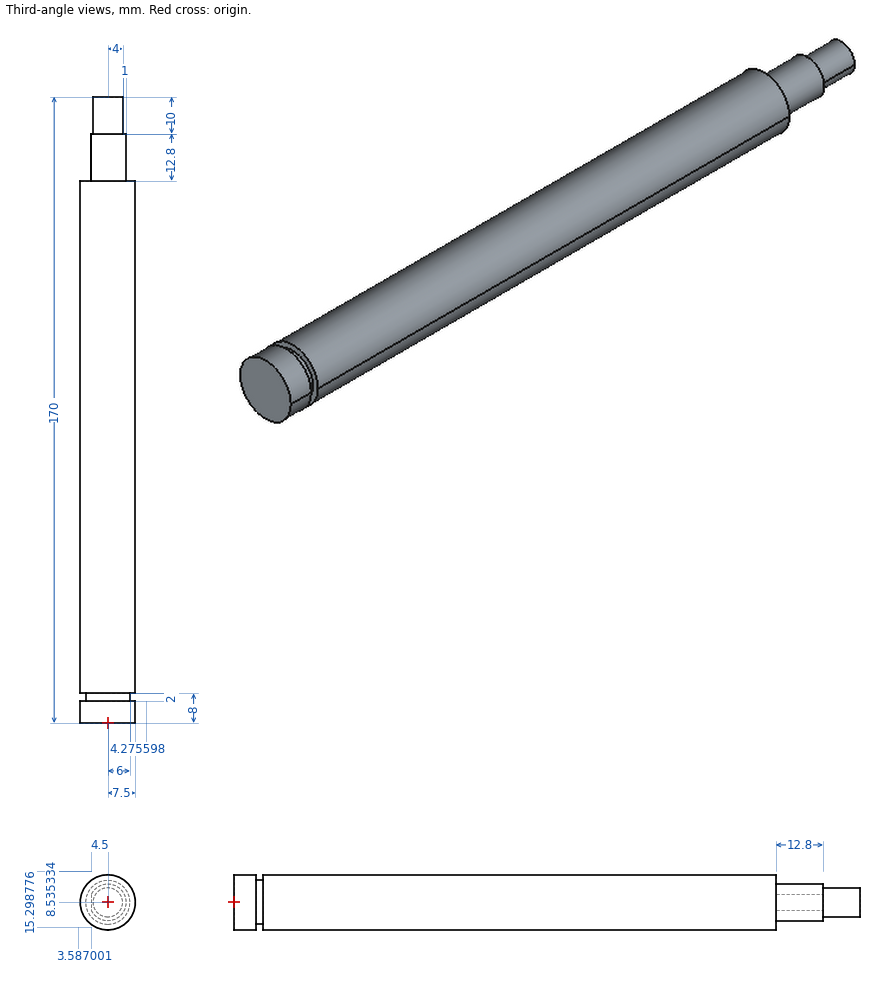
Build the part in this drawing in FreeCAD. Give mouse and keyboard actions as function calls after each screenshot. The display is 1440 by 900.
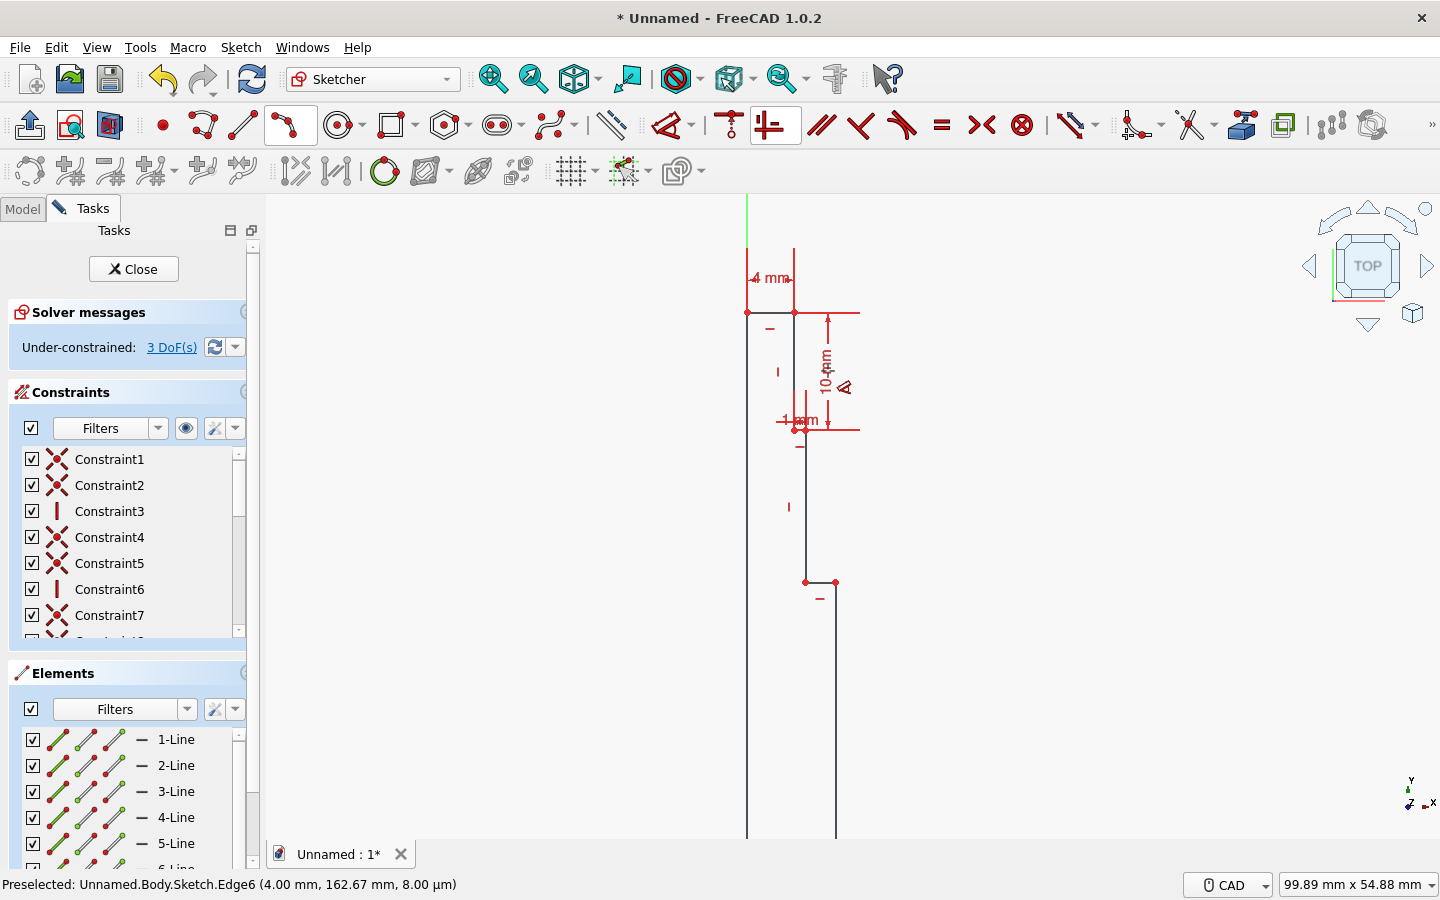
scroll(783, 316, down, 8)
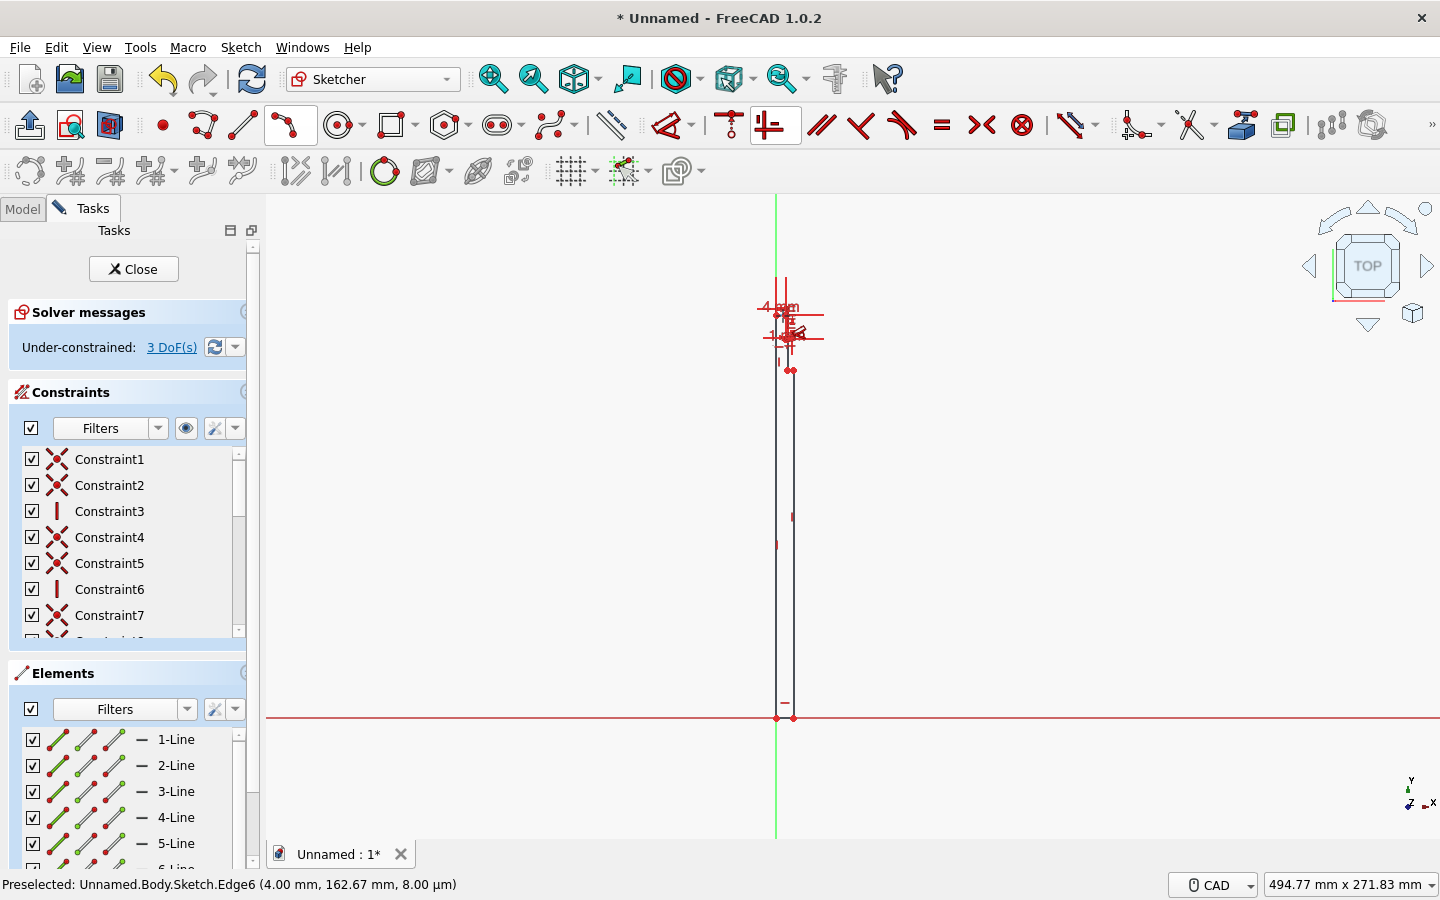
scroll(781, 718, up, 5)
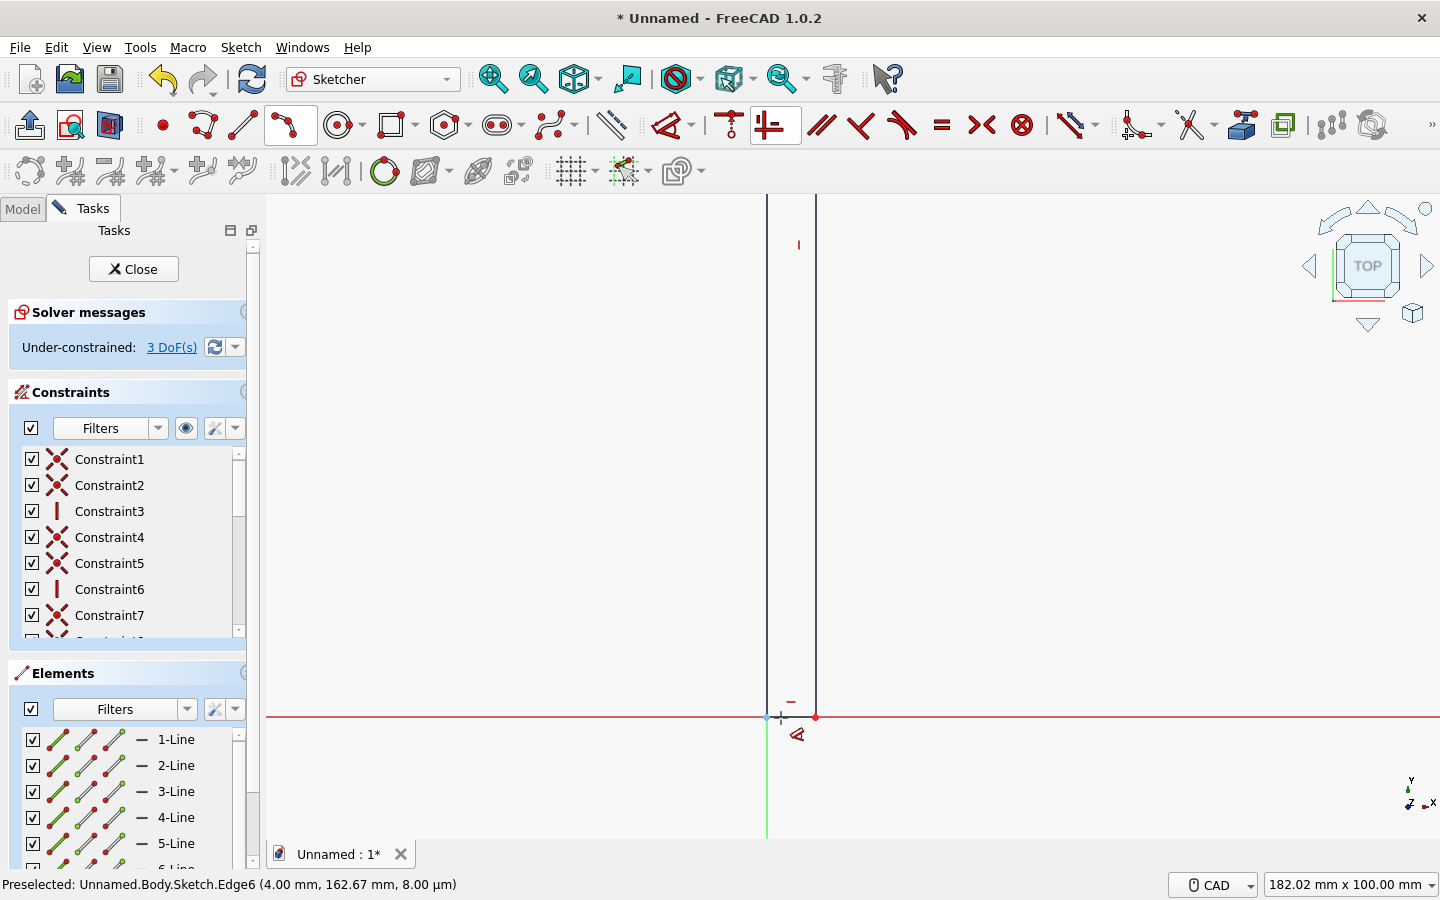
click(782, 717)
click(791, 751)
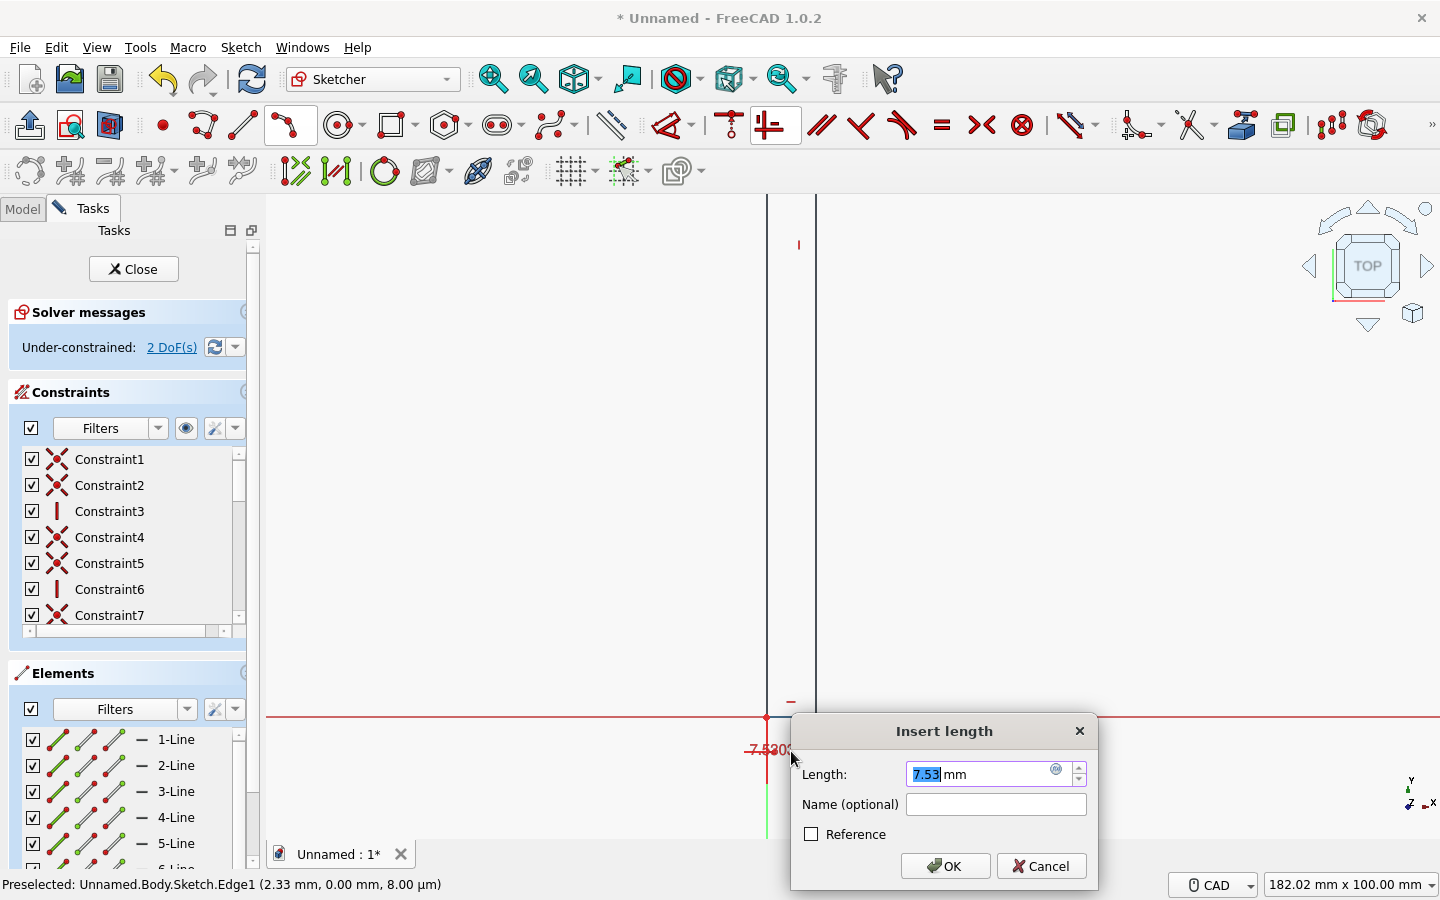
text(7.5)
key(Return)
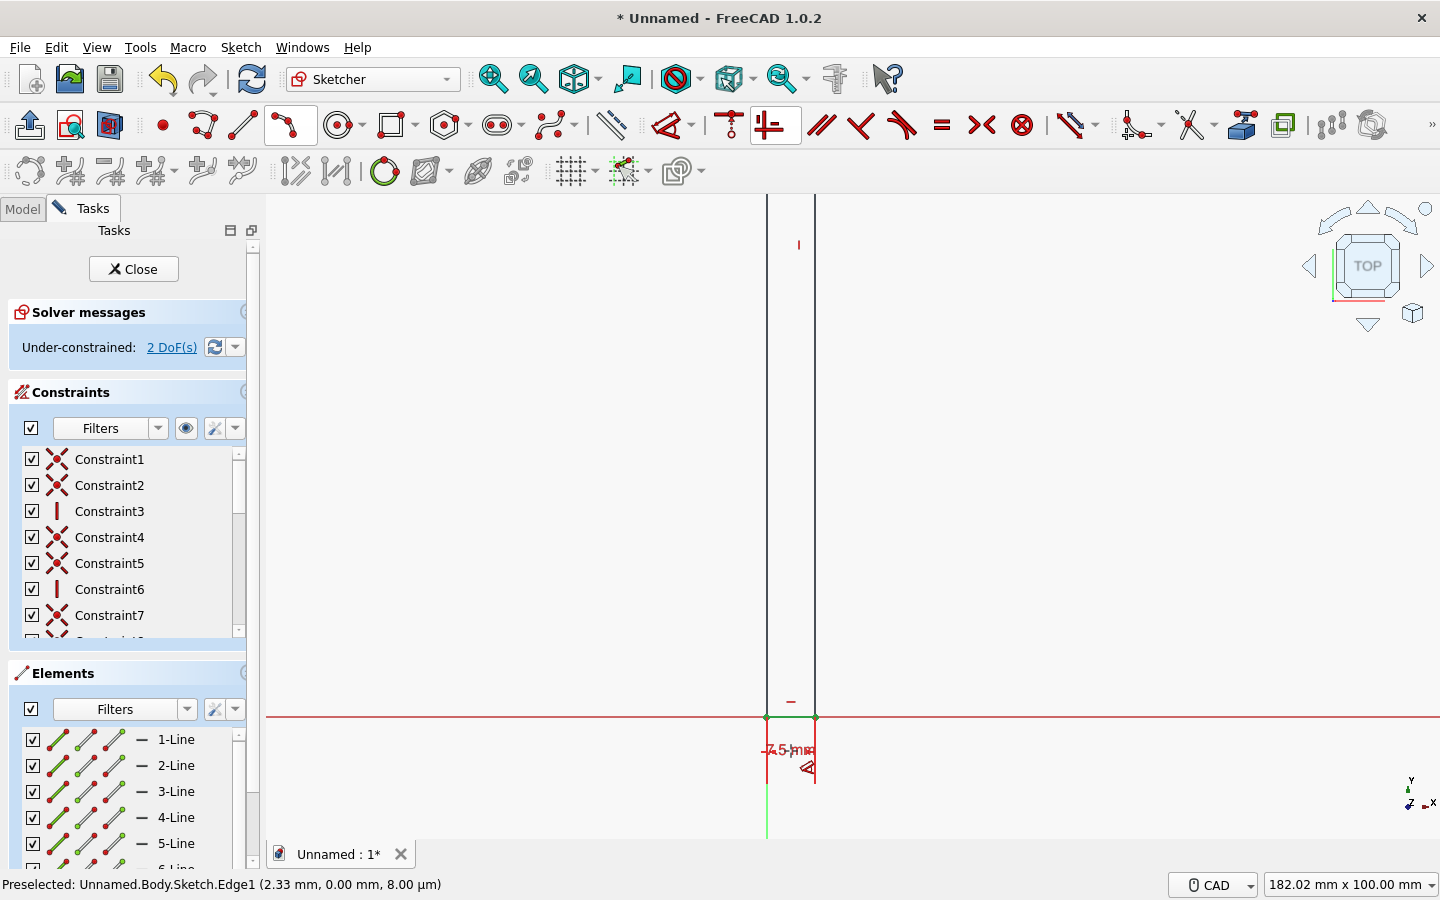
click(767, 389)
click(733, 470)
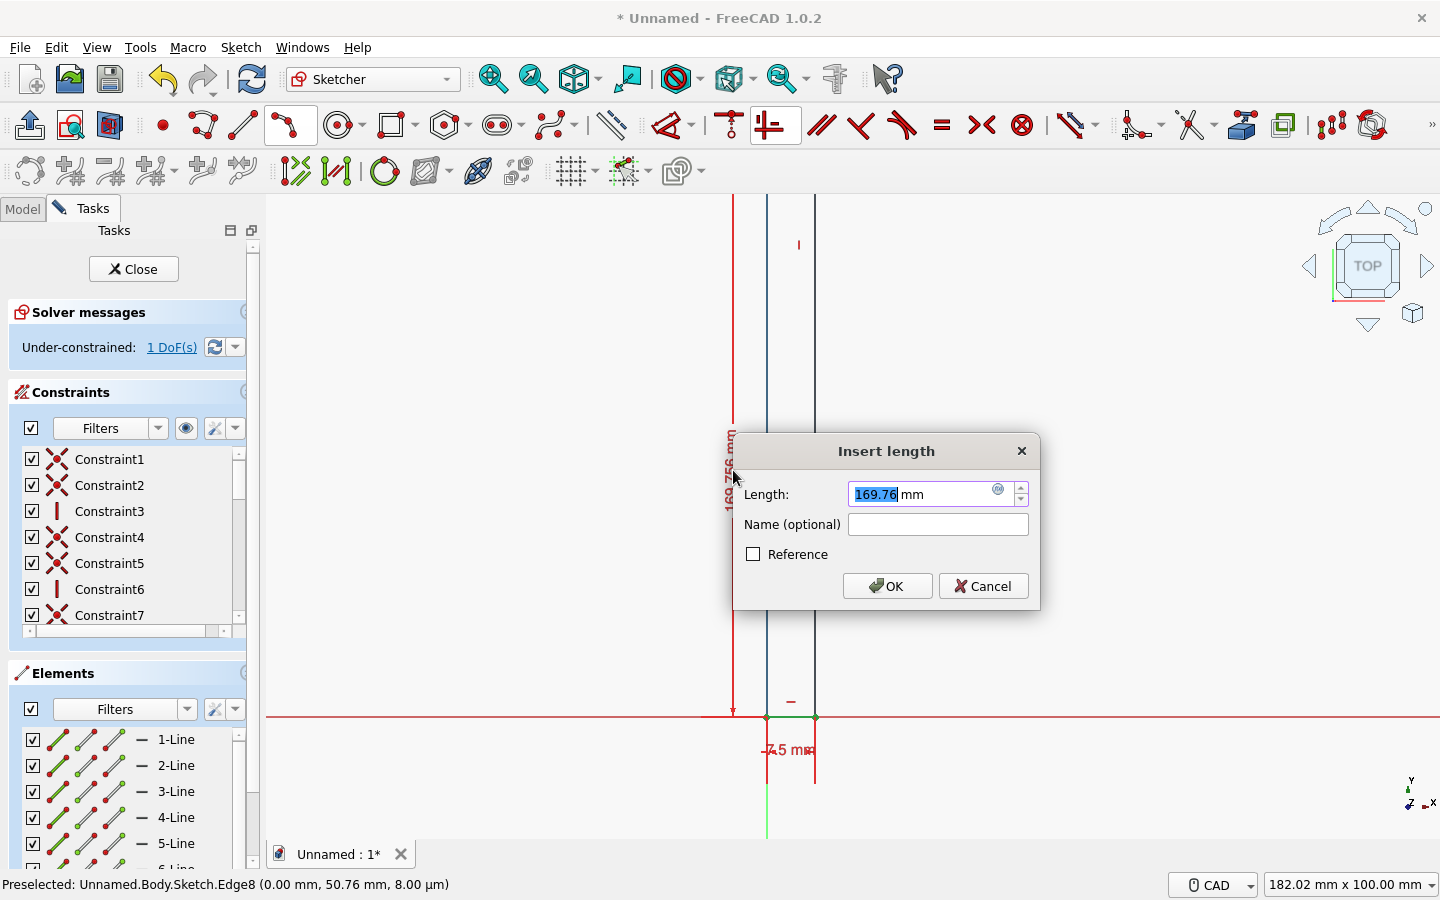
text(170)
key(Return)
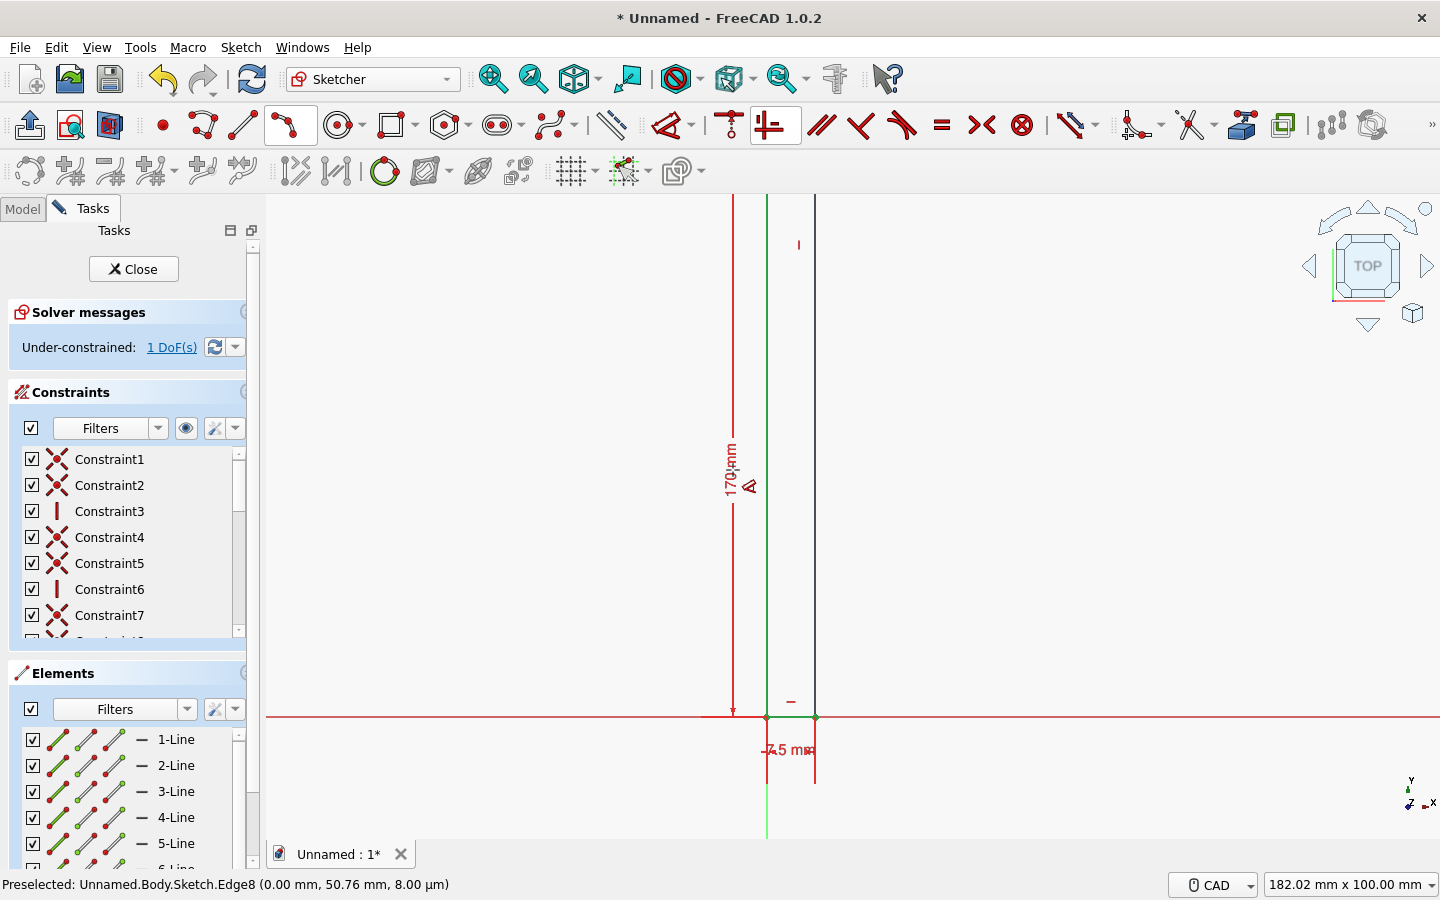
scroll(781, 719, down, 5)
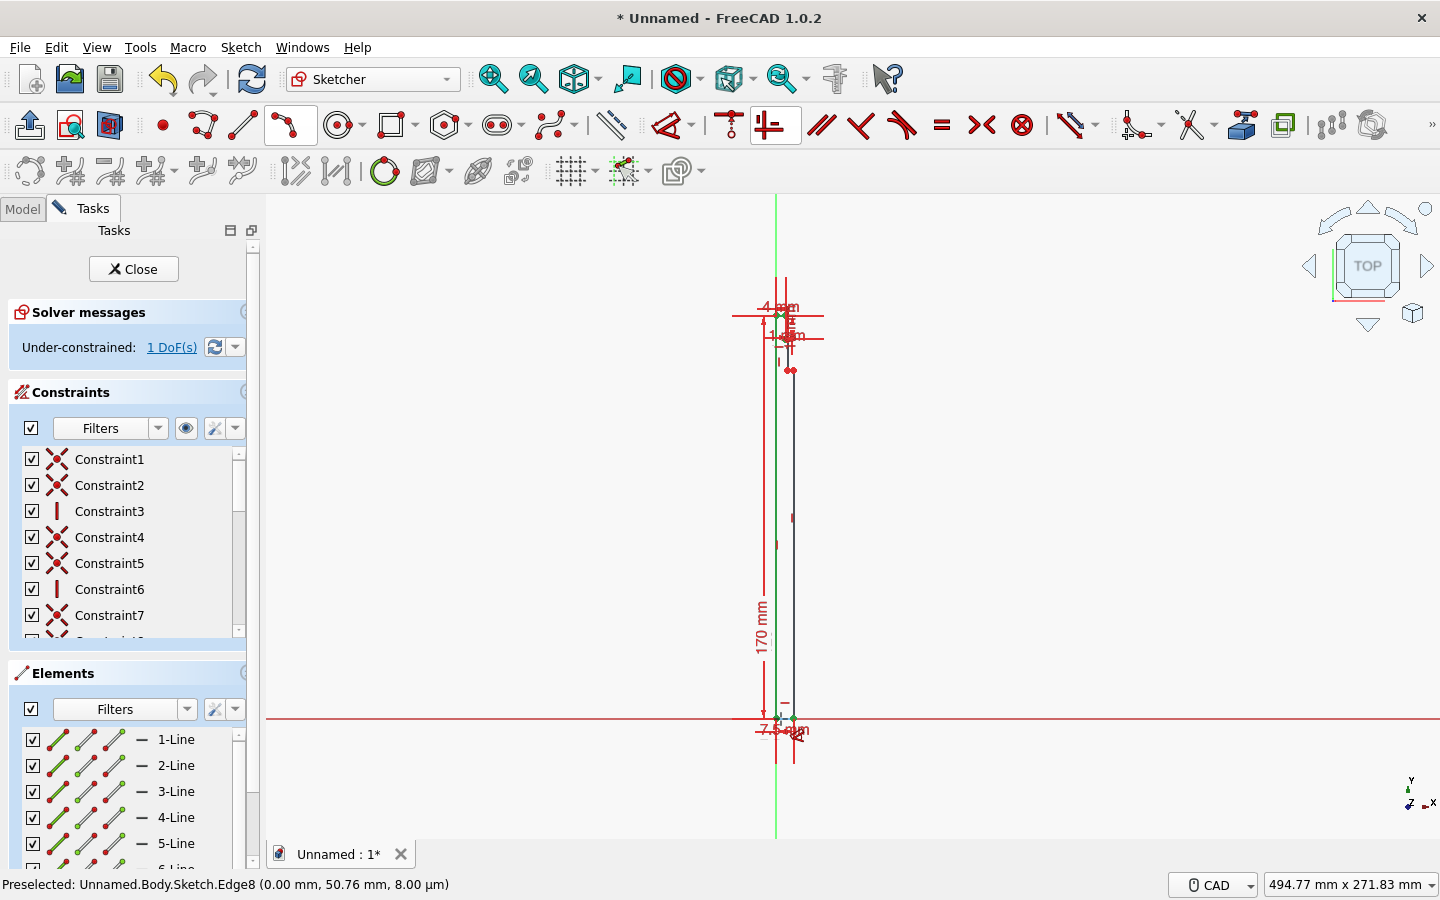
scroll(788, 361, up, 2)